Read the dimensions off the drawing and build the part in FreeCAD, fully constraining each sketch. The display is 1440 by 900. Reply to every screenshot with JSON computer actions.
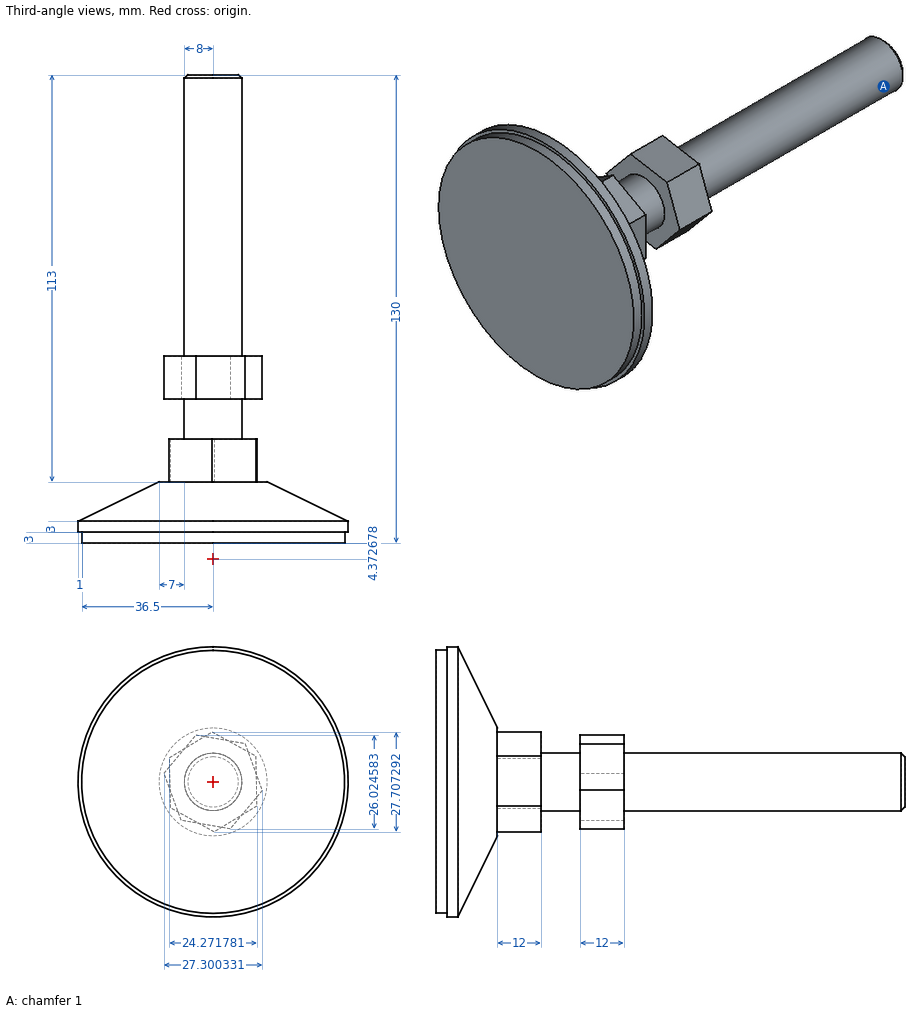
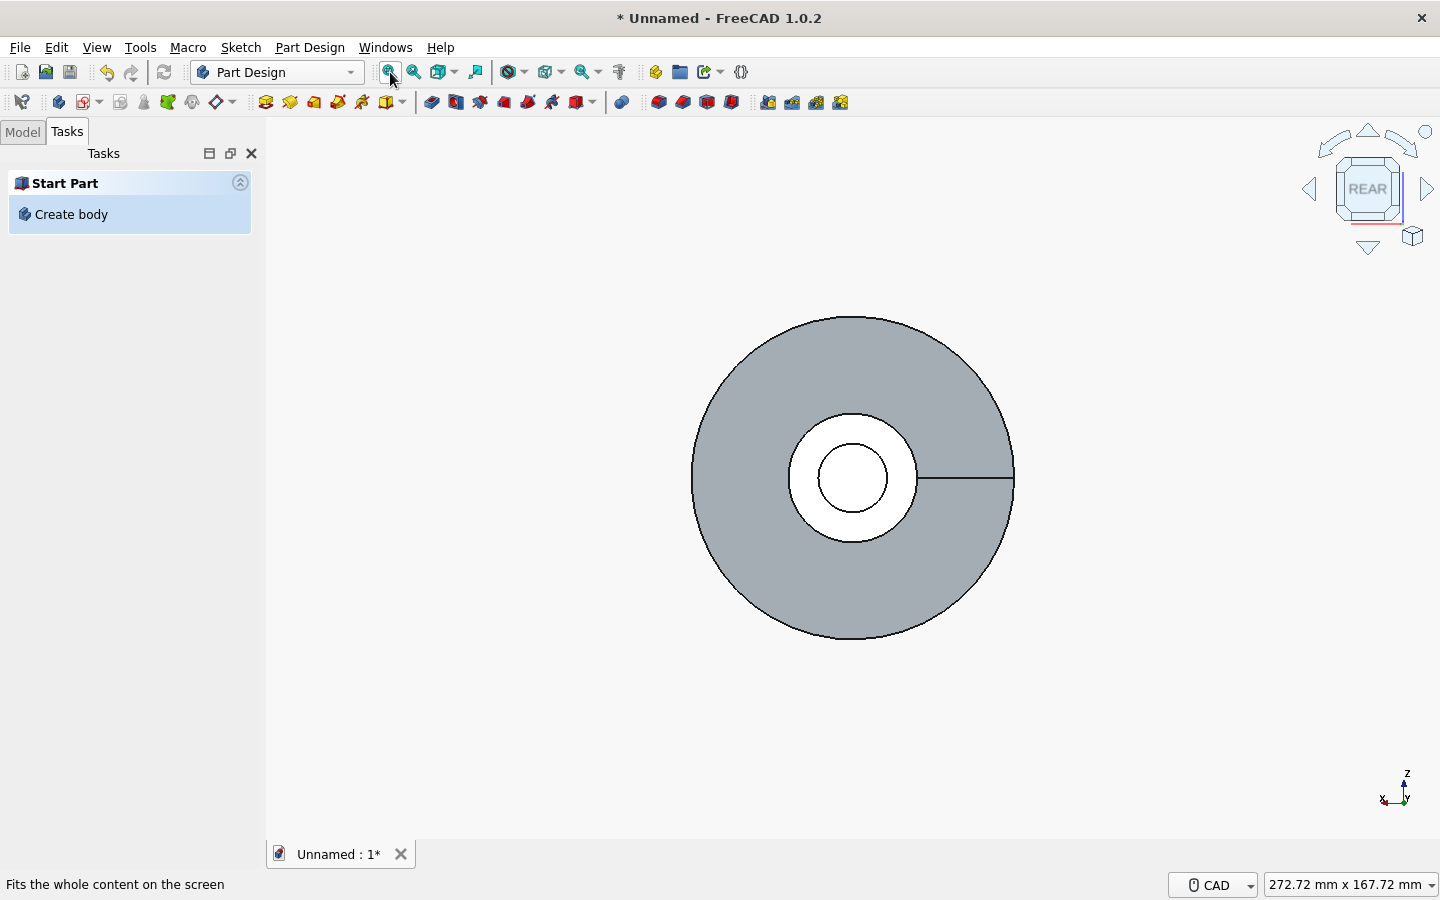
{"action": "left_click", "coordinate": [890, 514]}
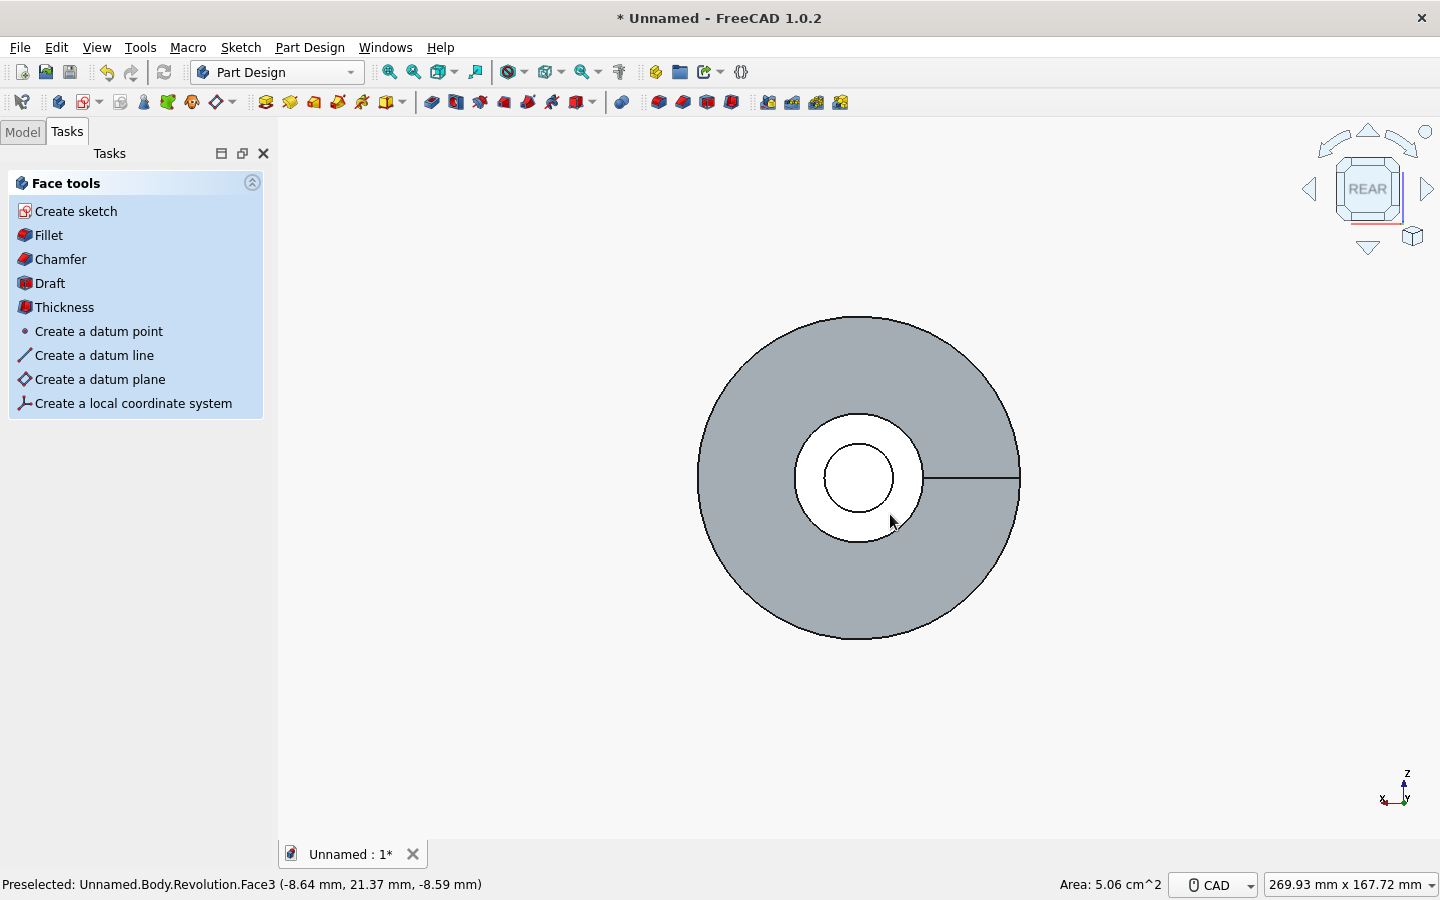
{"action": "left_click", "coordinate": [84, 102]}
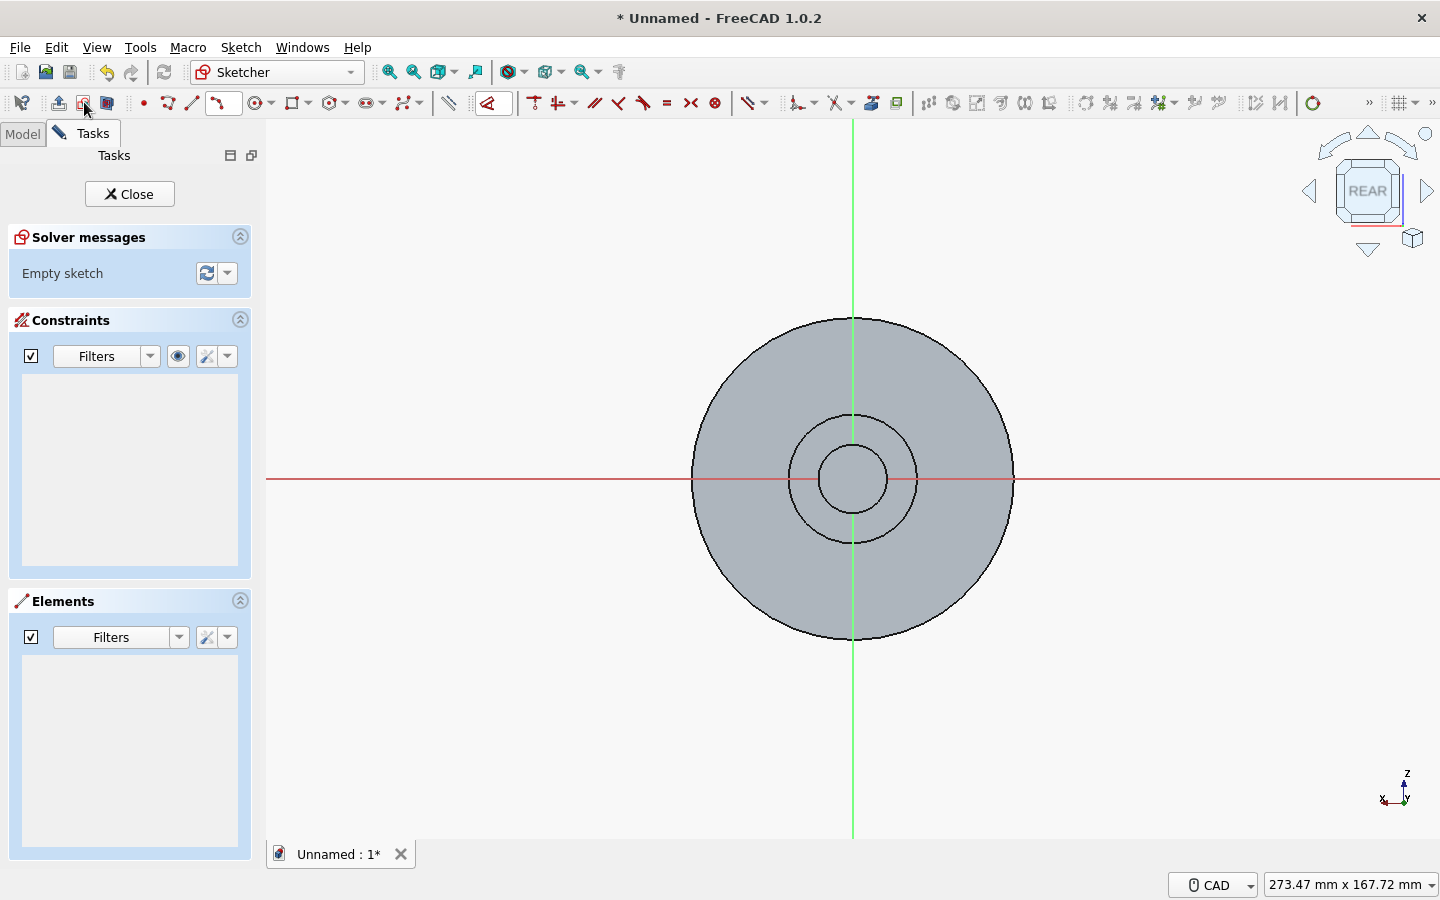
{"action": "left_click", "coordinate": [108, 104]}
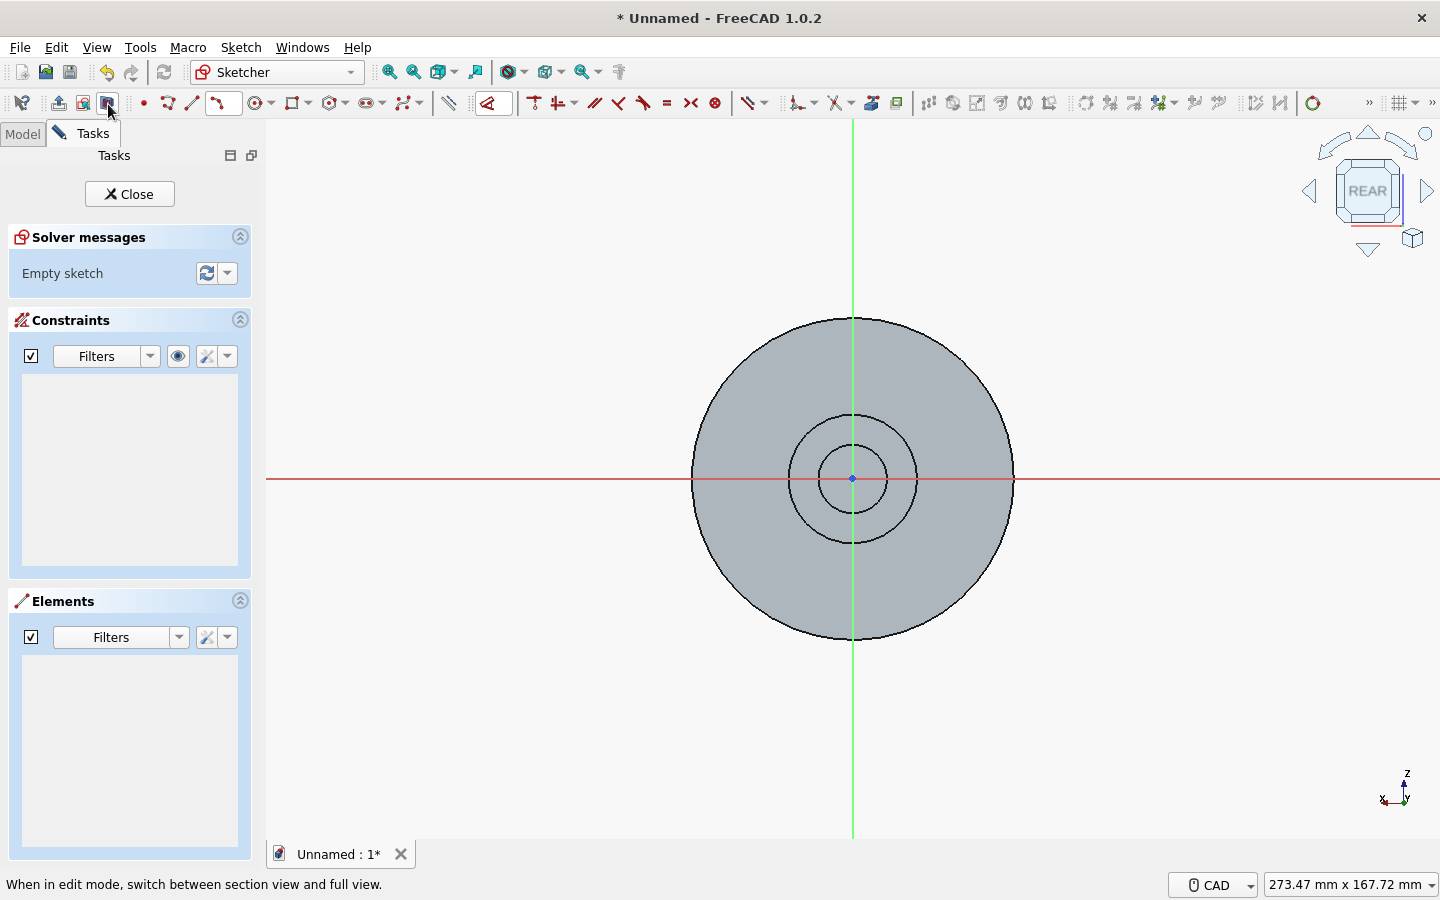
{"action": "scroll", "coordinate": [875, 479], "scroll_direction": "up", "scroll_amount": 7}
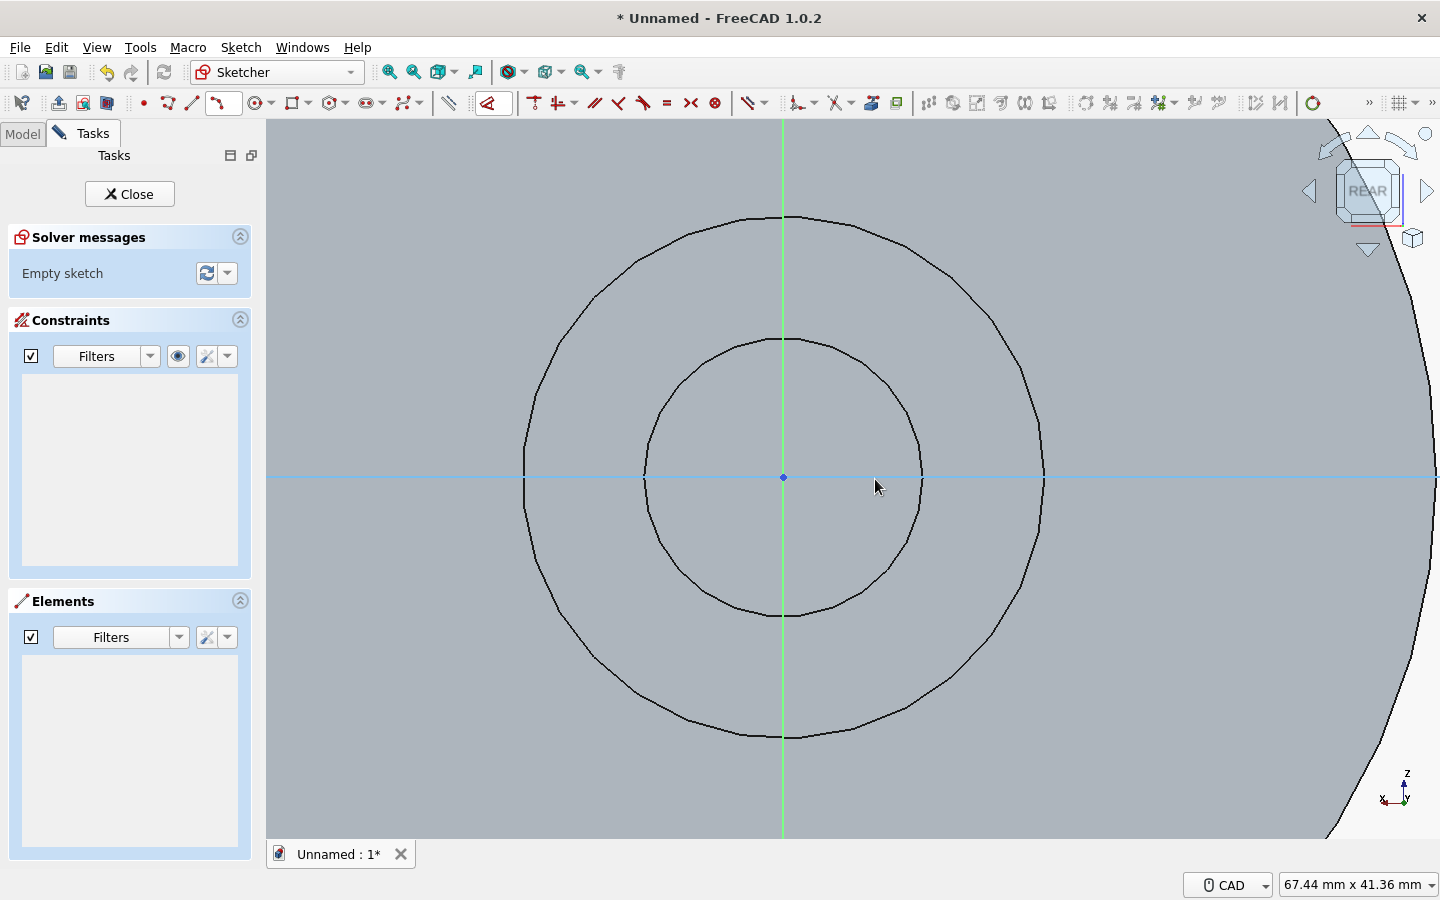
{"action": "left_click", "coordinate": [330, 104]}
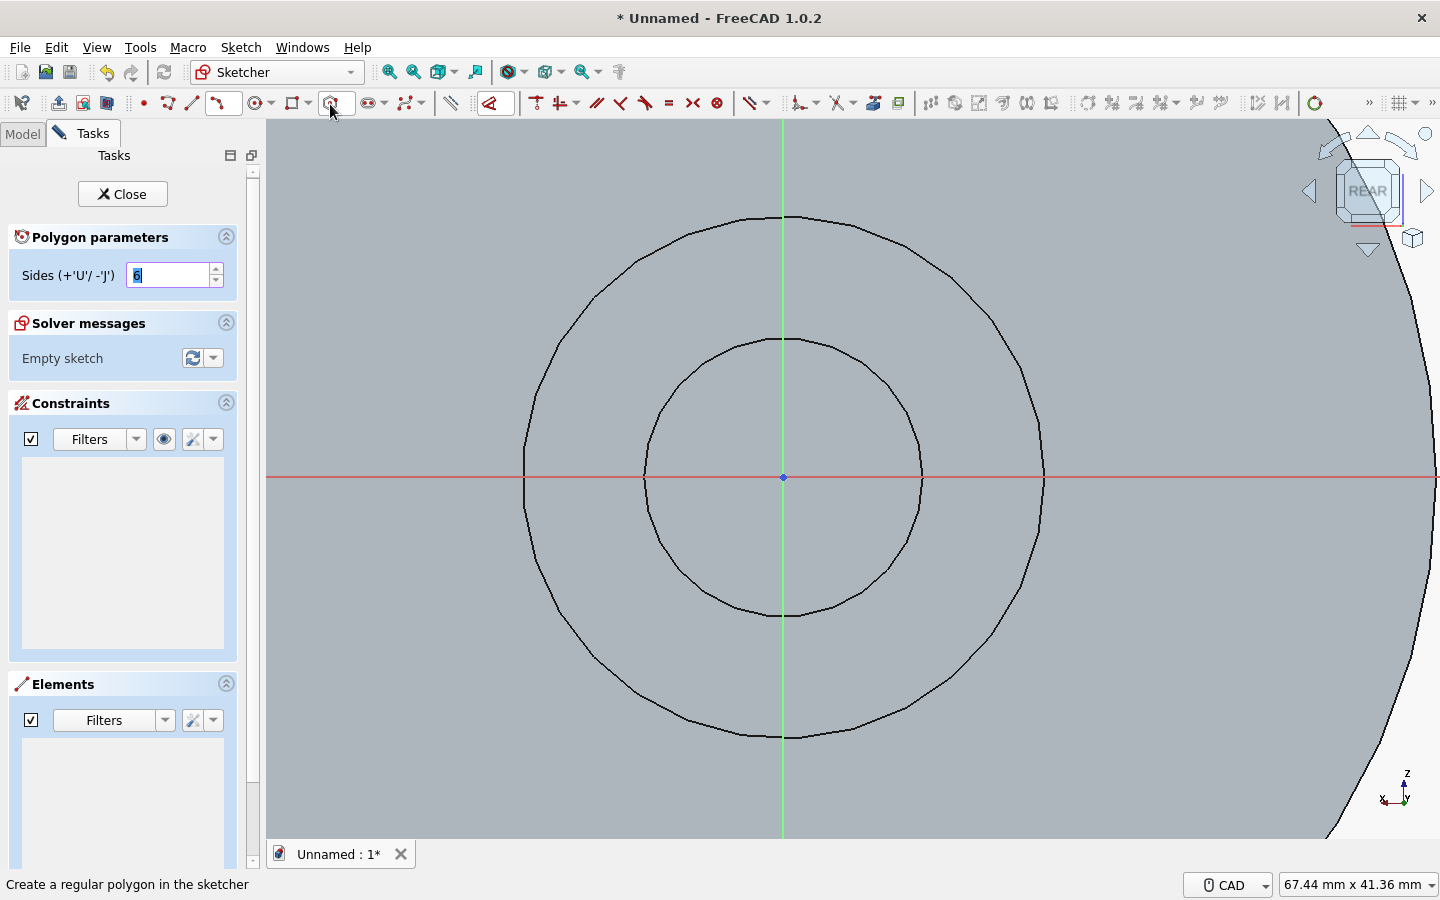
{"action": "left_click", "coordinate": [783, 477]}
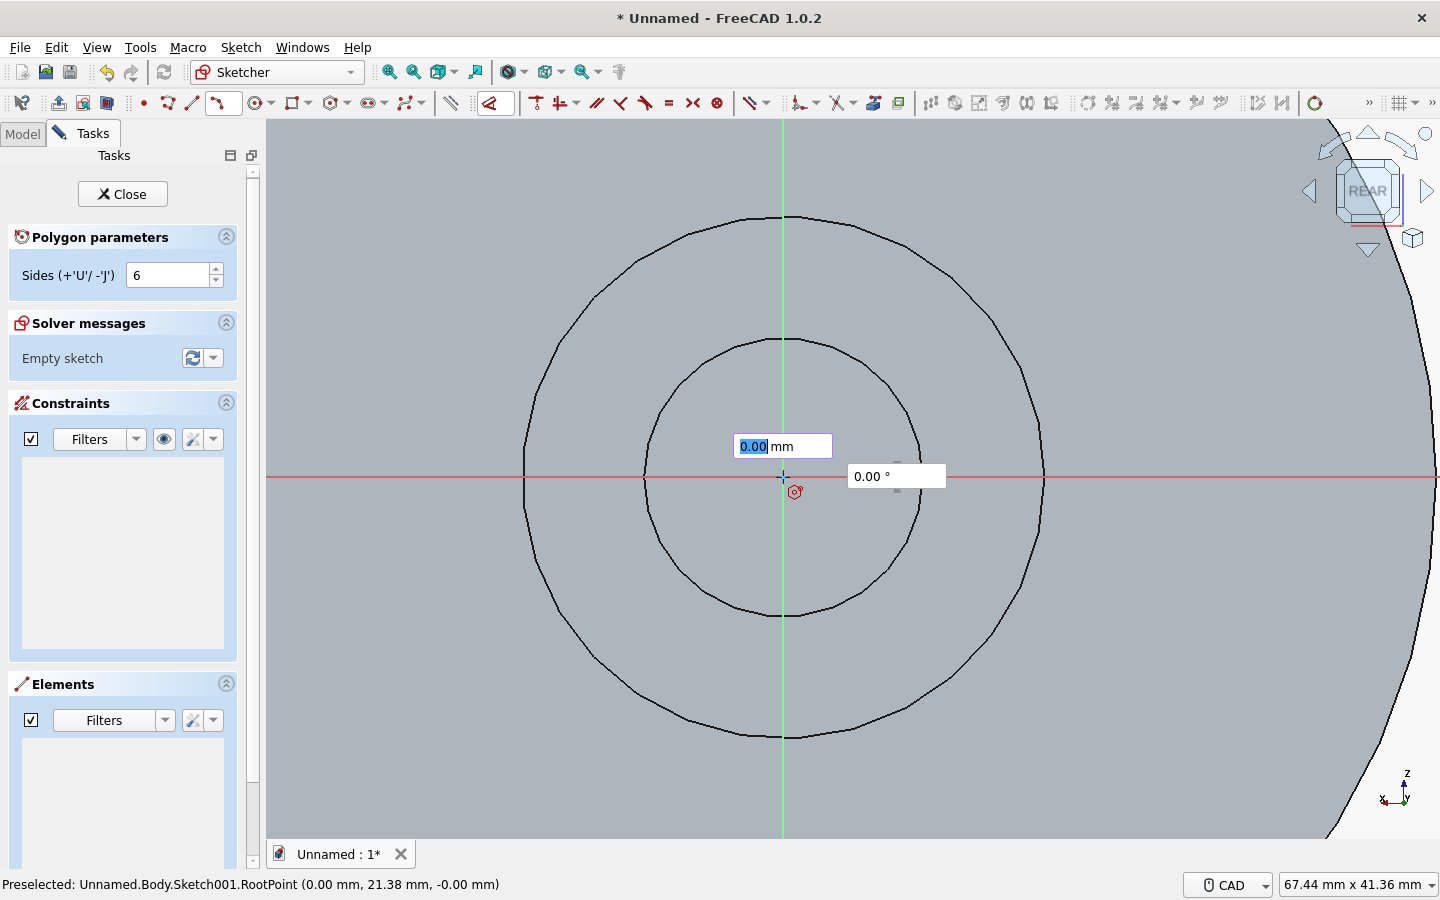
{"action": "left_click", "coordinate": [577, 353]}
{"action": "right_click", "coordinate": [577, 353]}